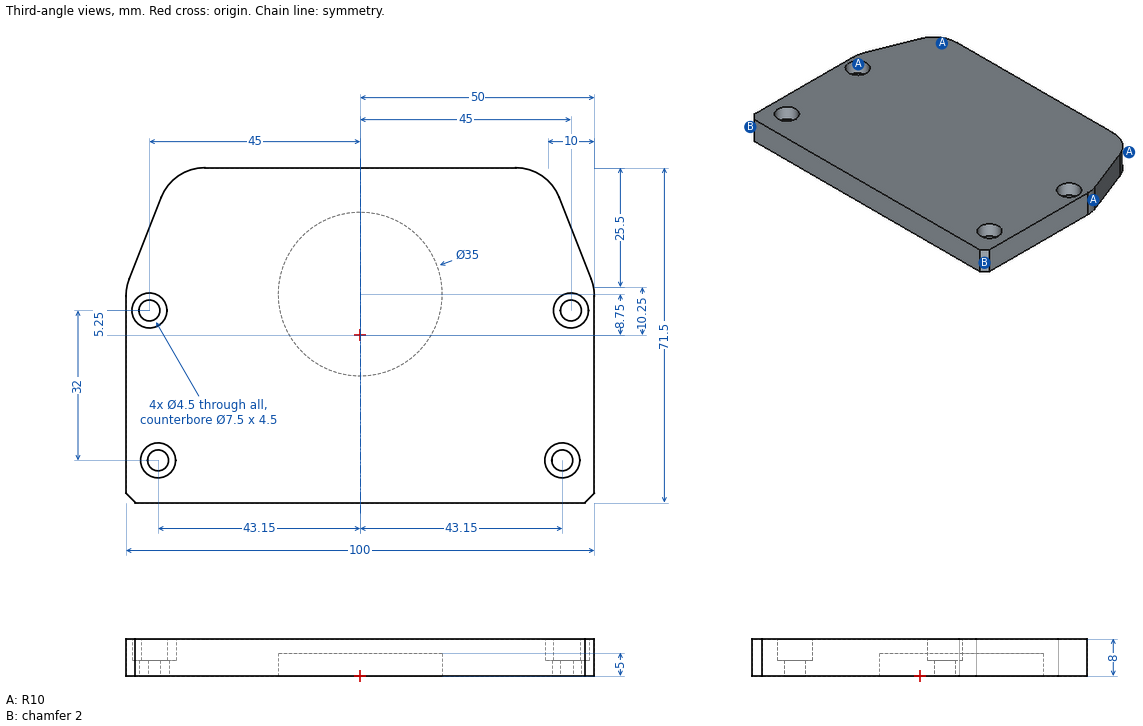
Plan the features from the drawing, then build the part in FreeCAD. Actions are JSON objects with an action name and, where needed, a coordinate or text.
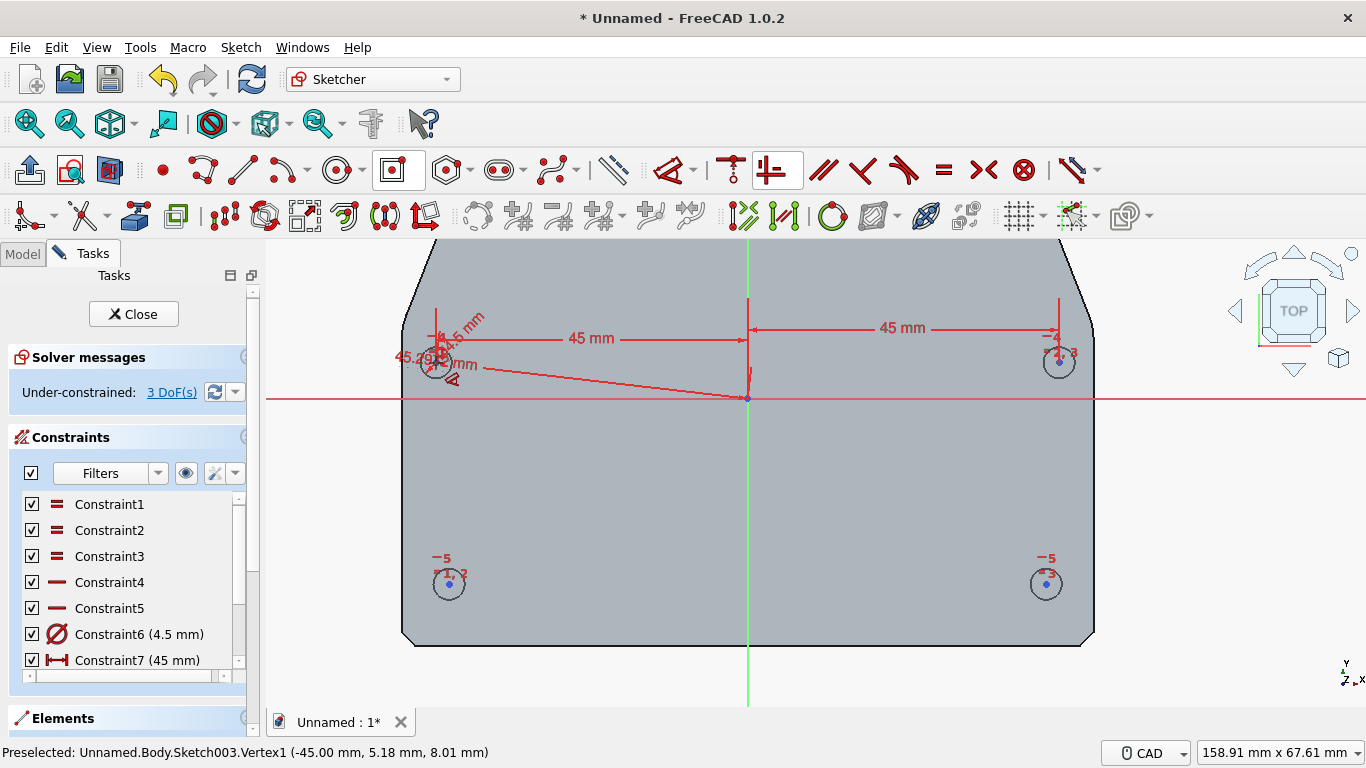
{"action": "left_click", "coordinate": [449, 584]}
{"action": "left_click", "coordinate": [402, 473]}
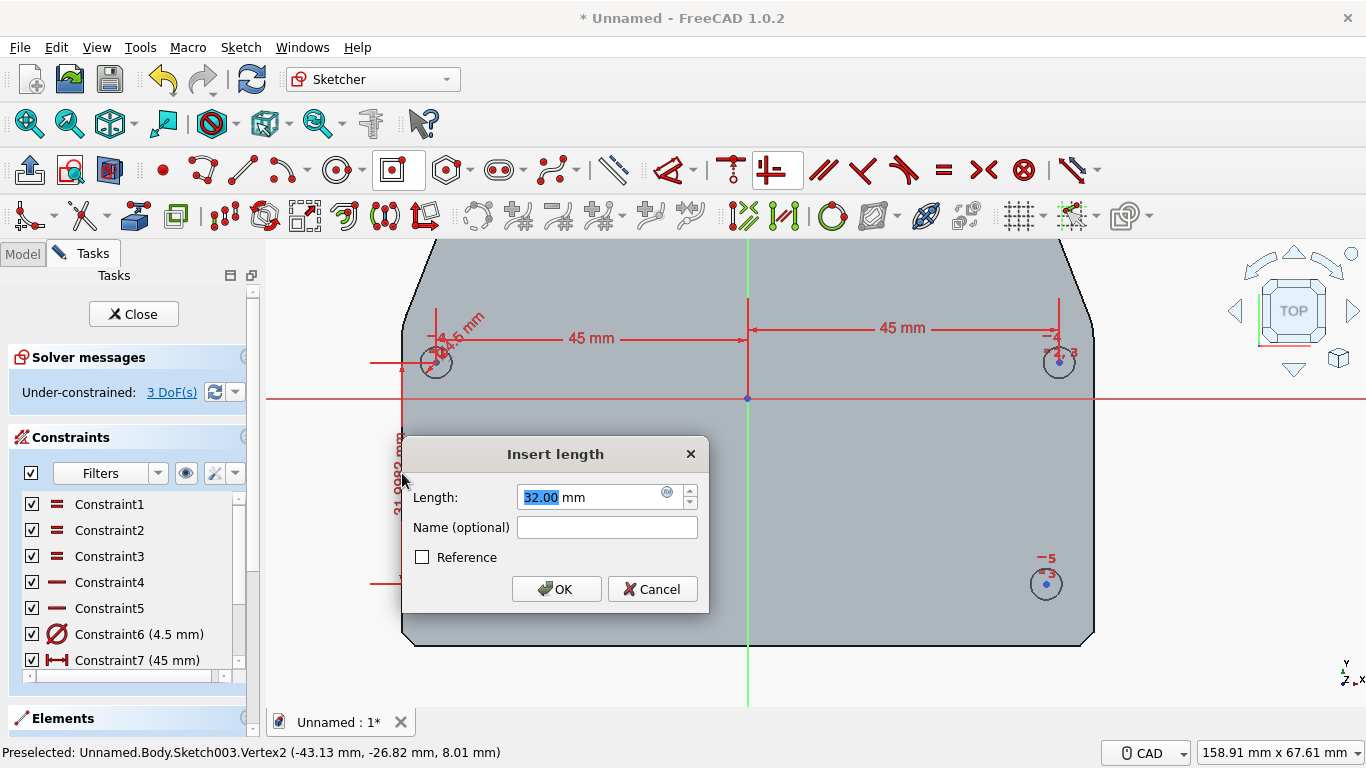
{"action": "type", "text": "32"}
{"action": "key", "text": "Return"}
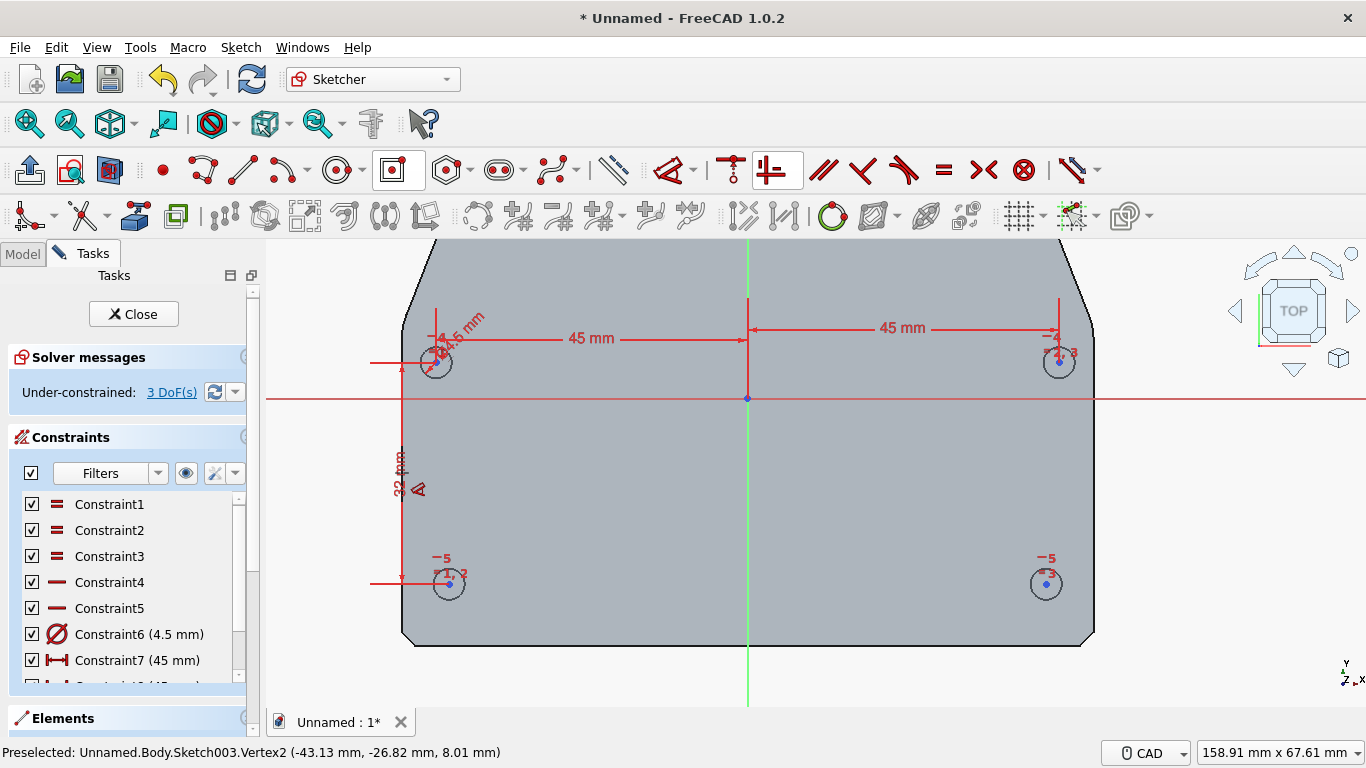
{"action": "left_click", "coordinate": [436, 363]}
{"action": "left_click", "coordinate": [402, 381]}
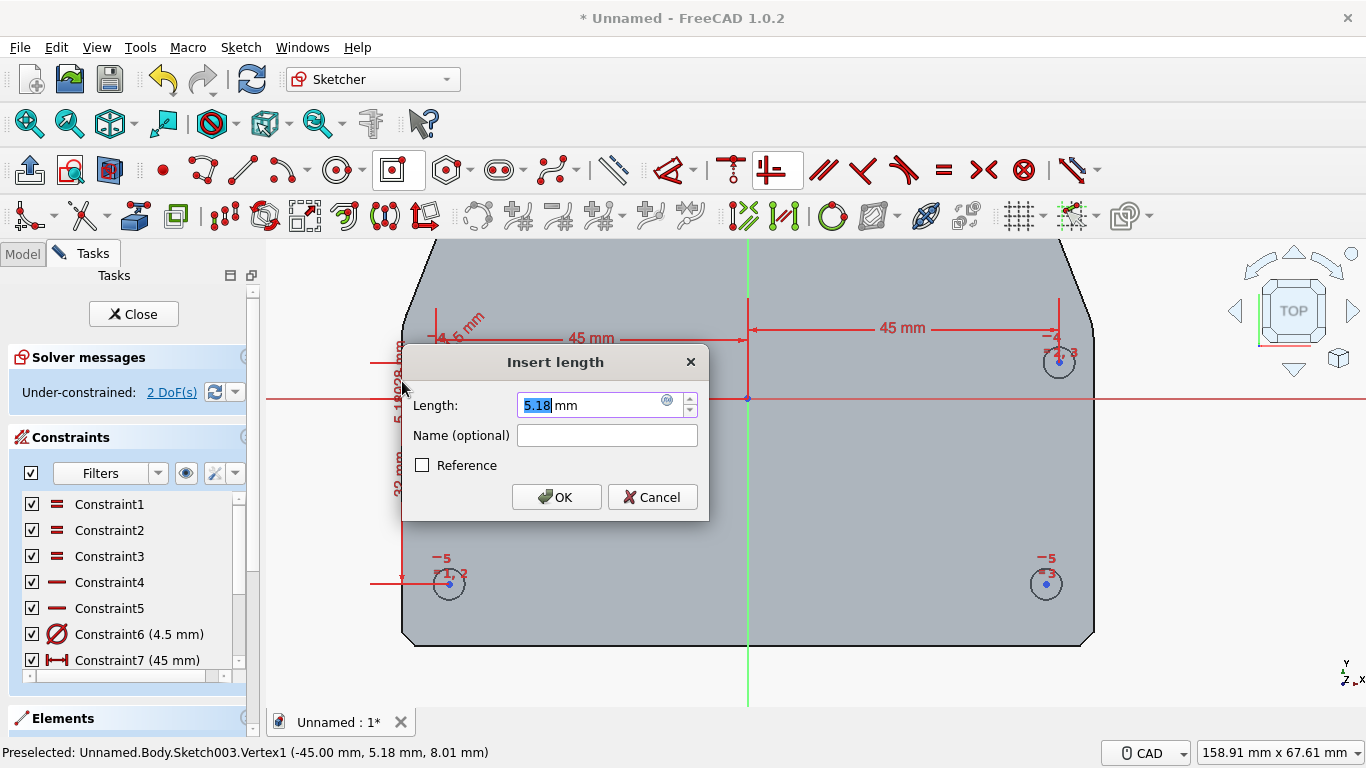
{"action": "type", "text": "5.25"}
{"action": "key", "text": "Return"}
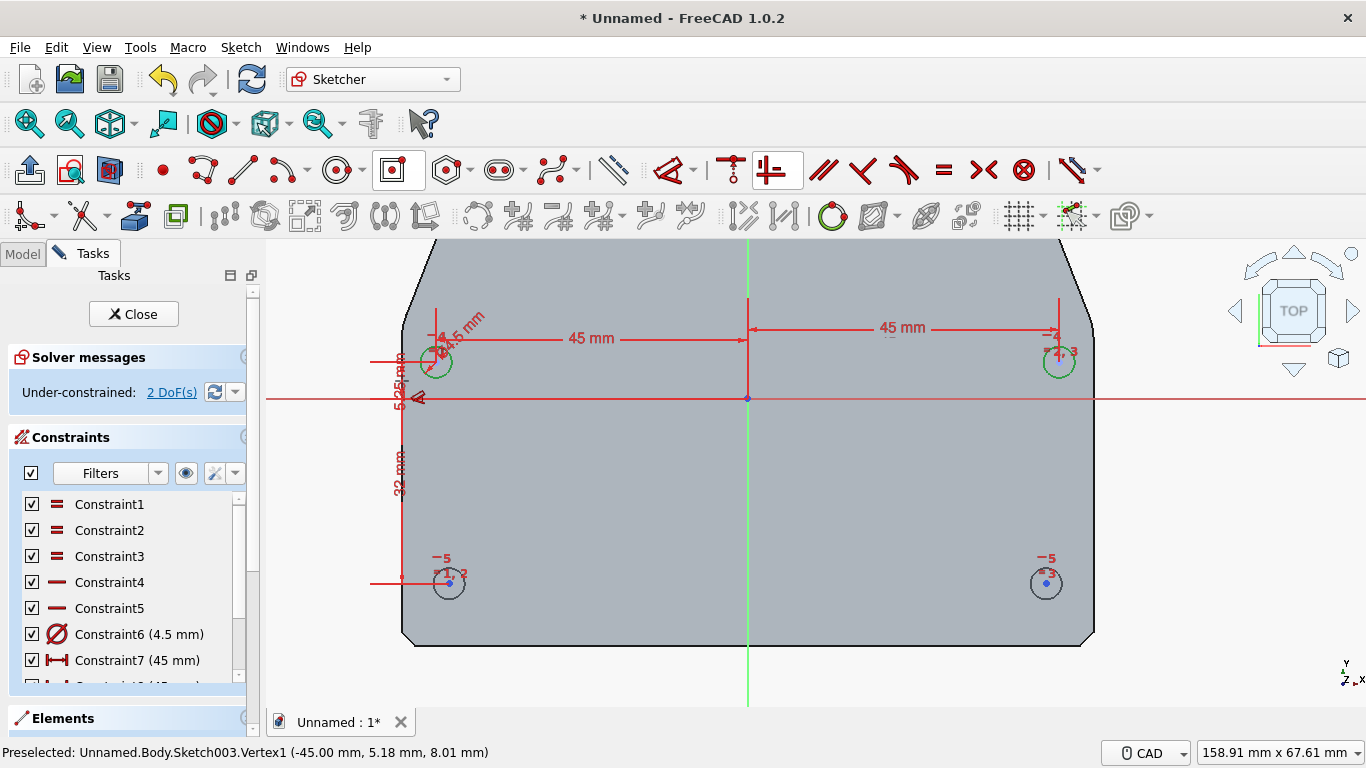
{"action": "left_click", "coordinate": [449, 584]}
{"action": "left_click", "coordinate": [598, 618]}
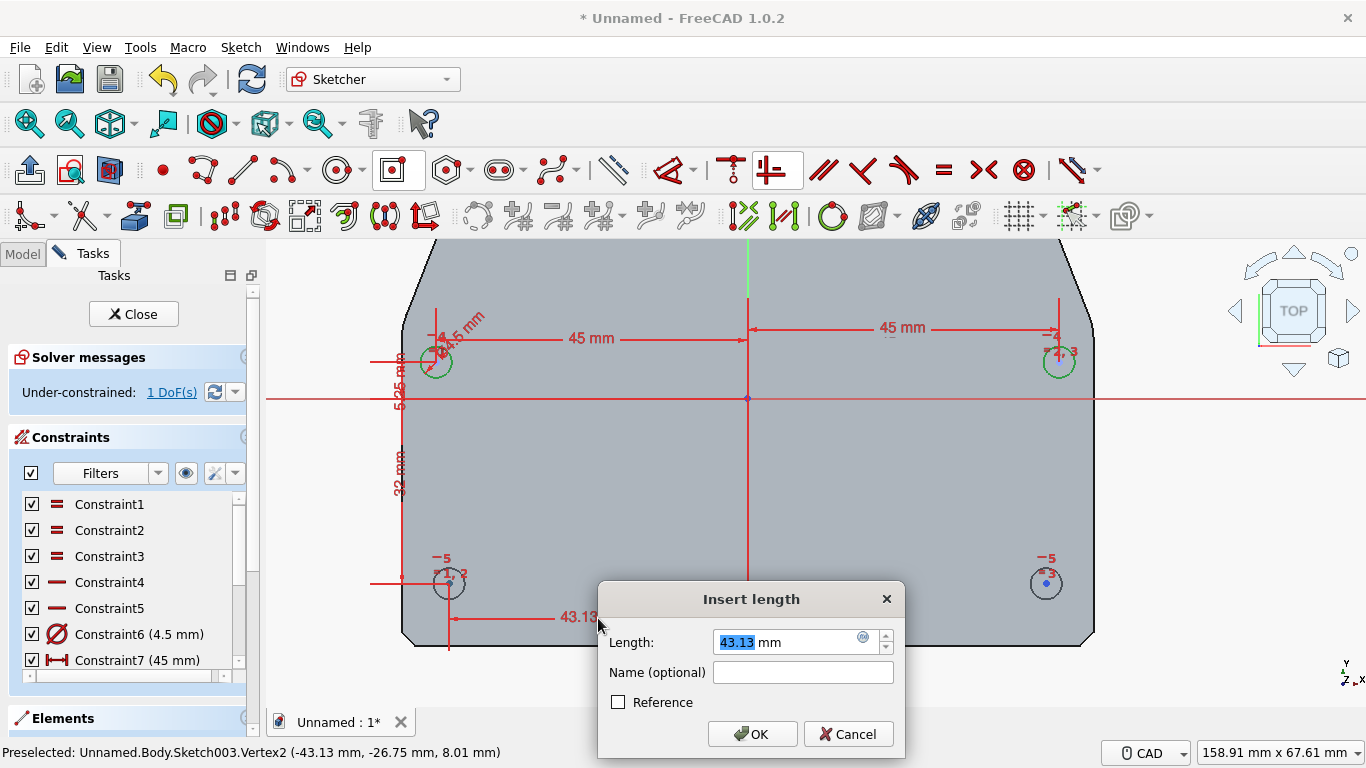
{"action": "type", "text": "43.15"}
{"action": "key", "text": "Return"}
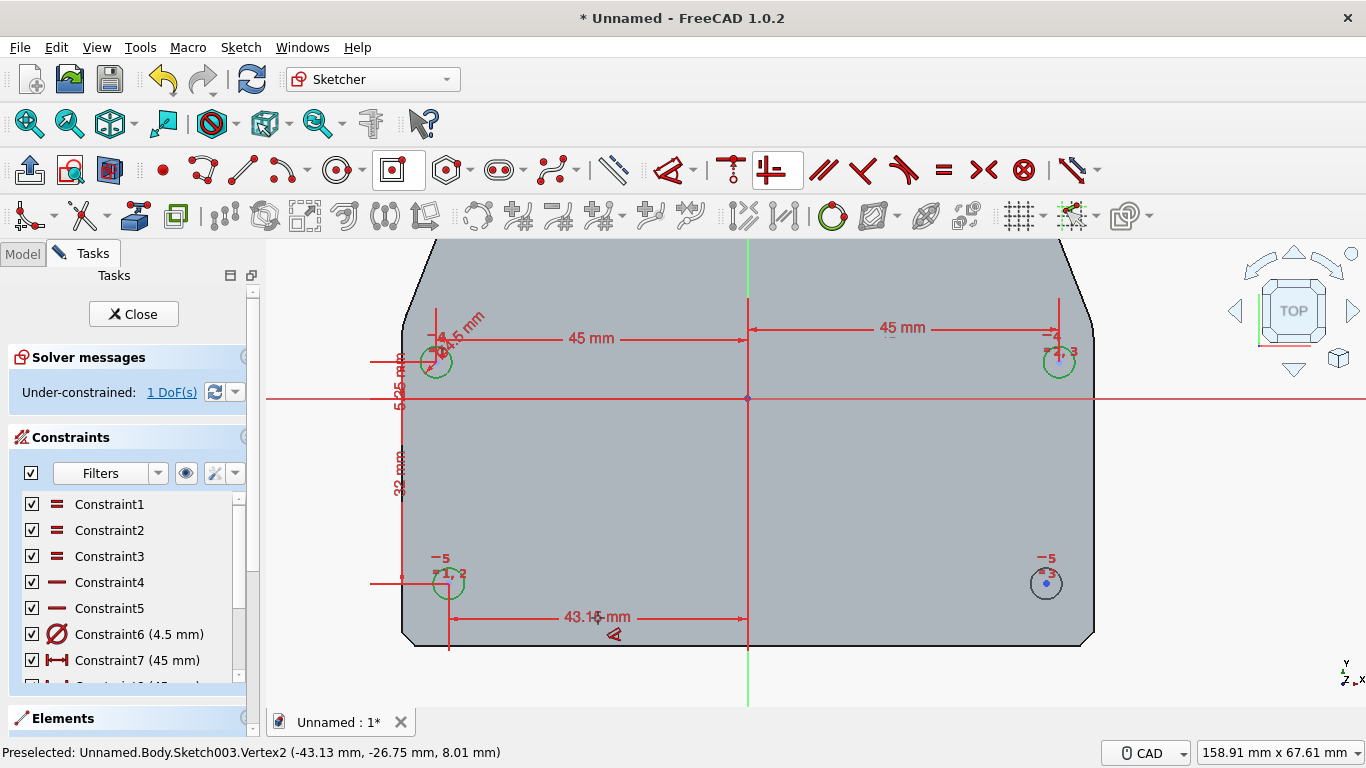
{"action": "left_click", "coordinate": [1046, 584]}
{"action": "left_click", "coordinate": [897, 618]}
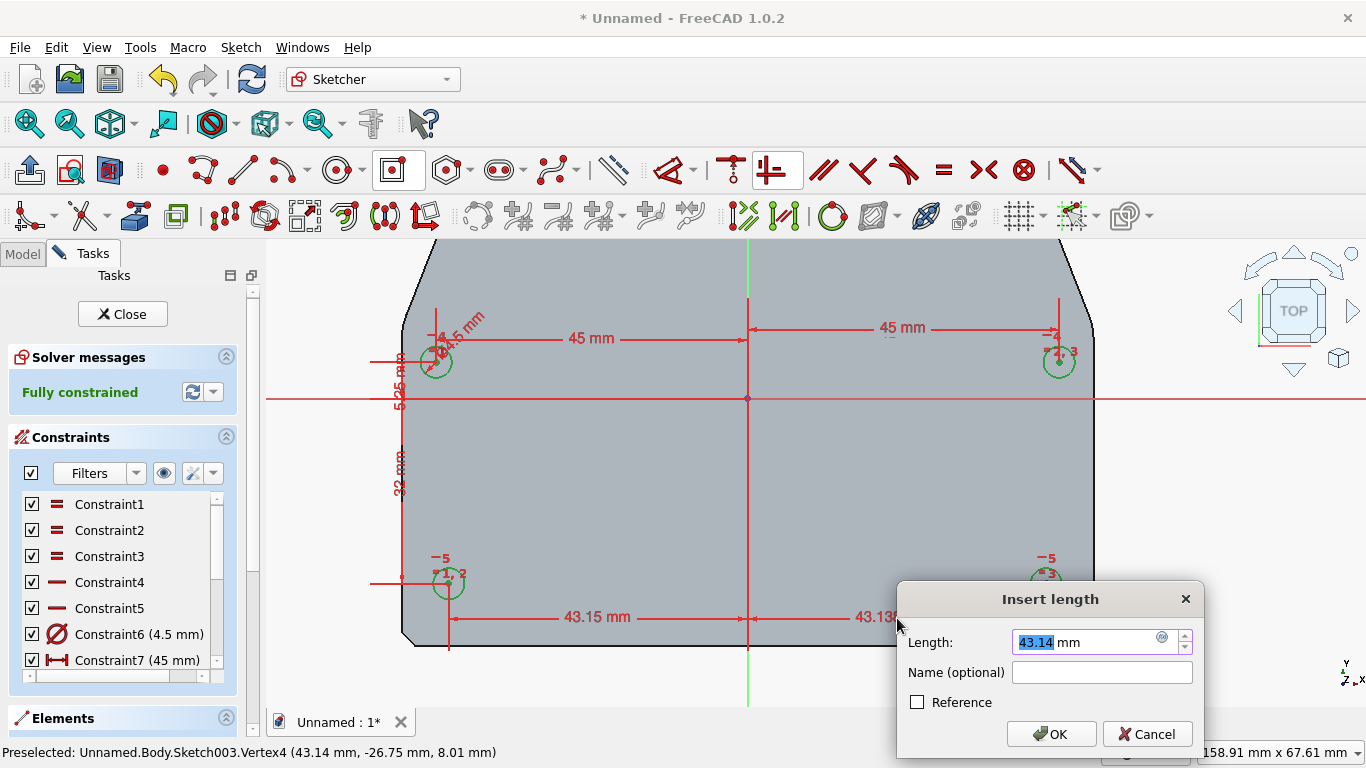
{"action": "type", "text": "43.15"}
{"action": "key", "text": "Return"}
{"action": "key", "text": "Escape"}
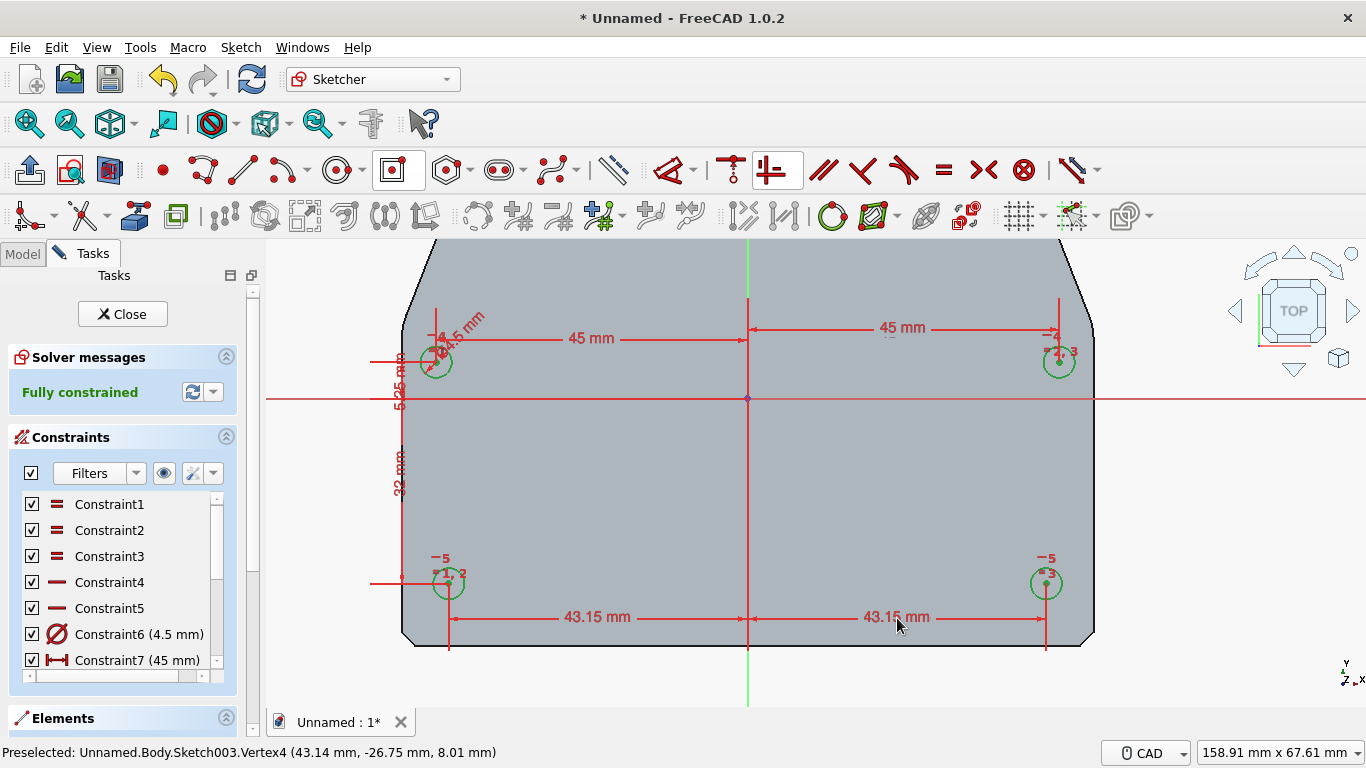
{"action": "left_click", "coordinate": [123, 314]}